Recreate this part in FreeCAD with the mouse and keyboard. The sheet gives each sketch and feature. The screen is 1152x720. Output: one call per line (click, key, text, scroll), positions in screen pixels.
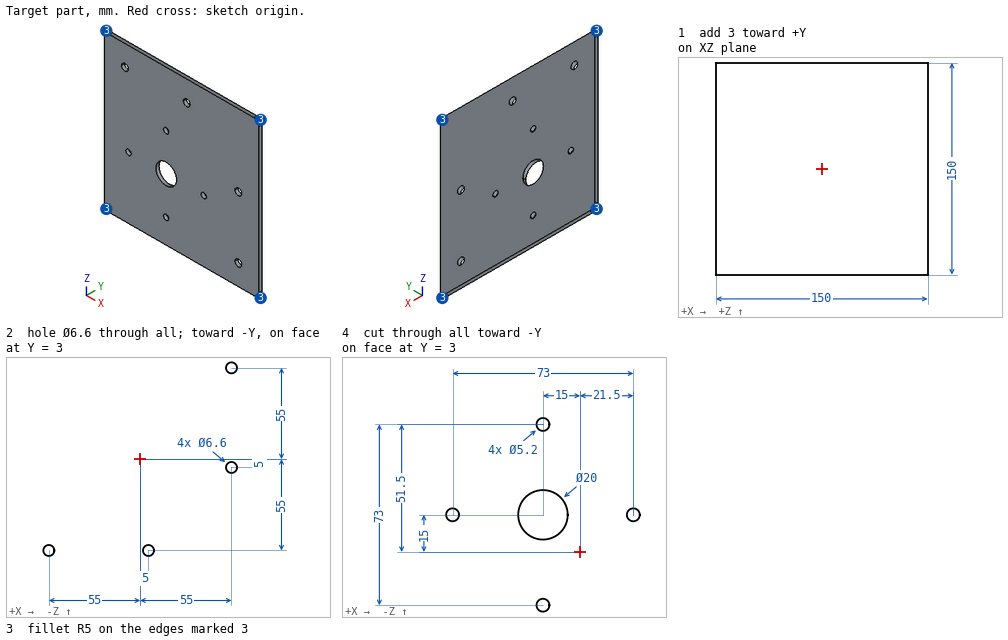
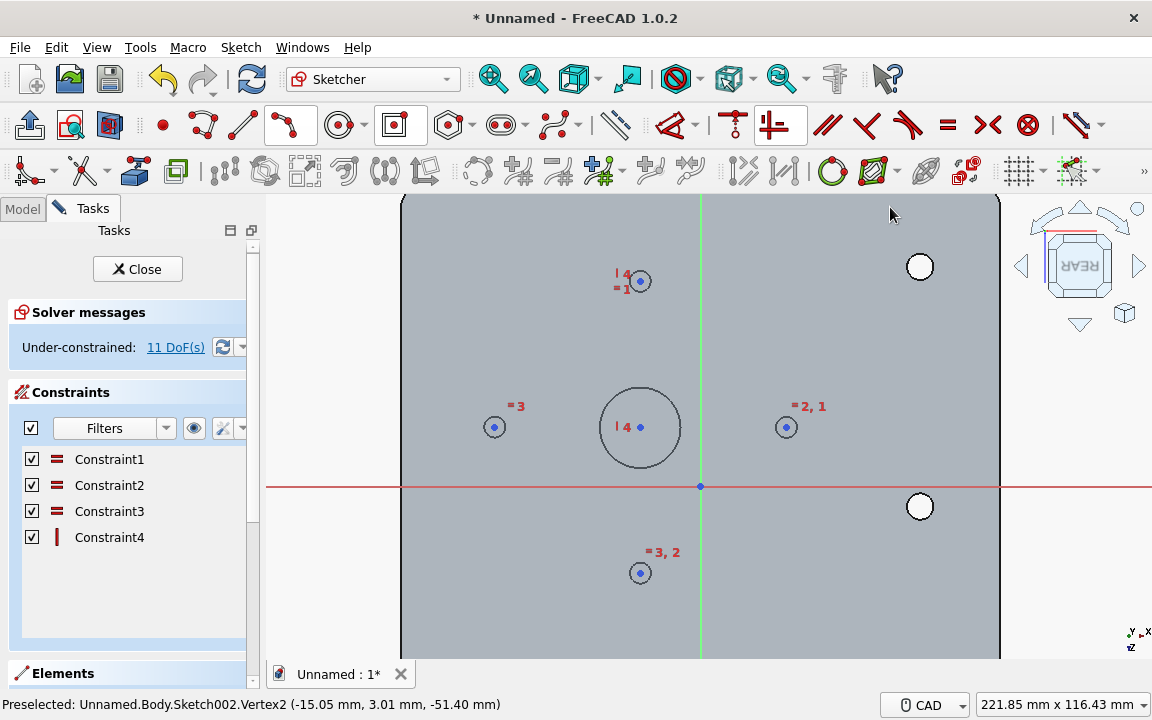
click(640, 428)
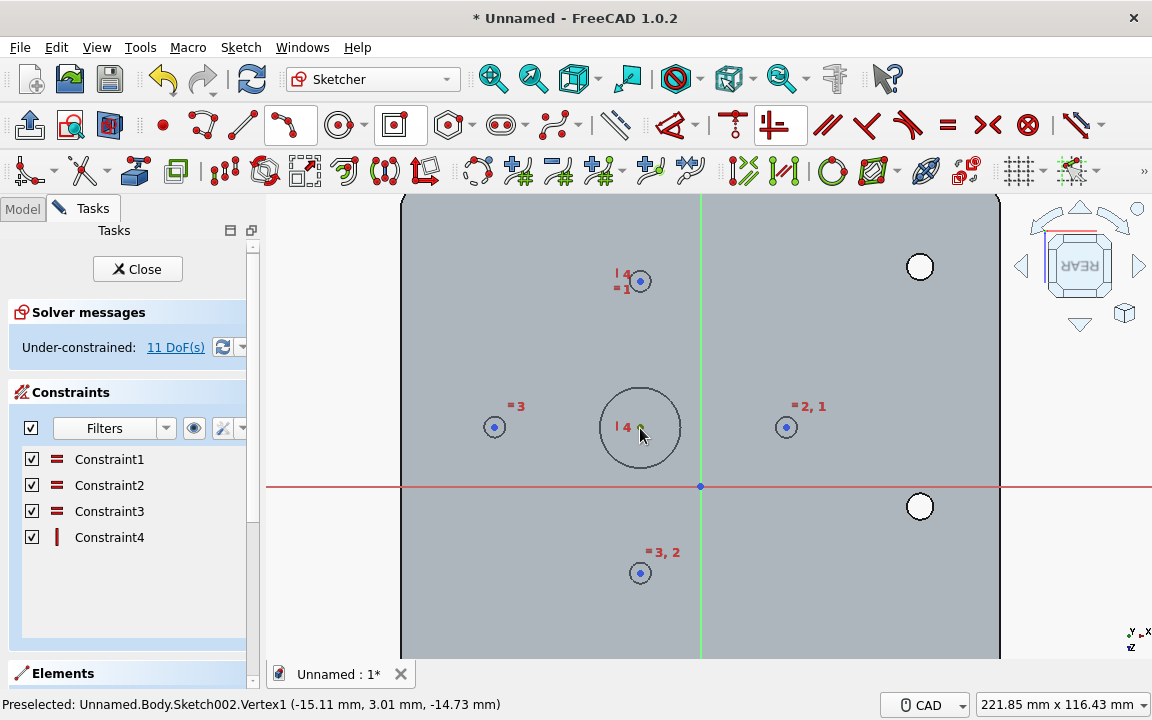
click(786, 427)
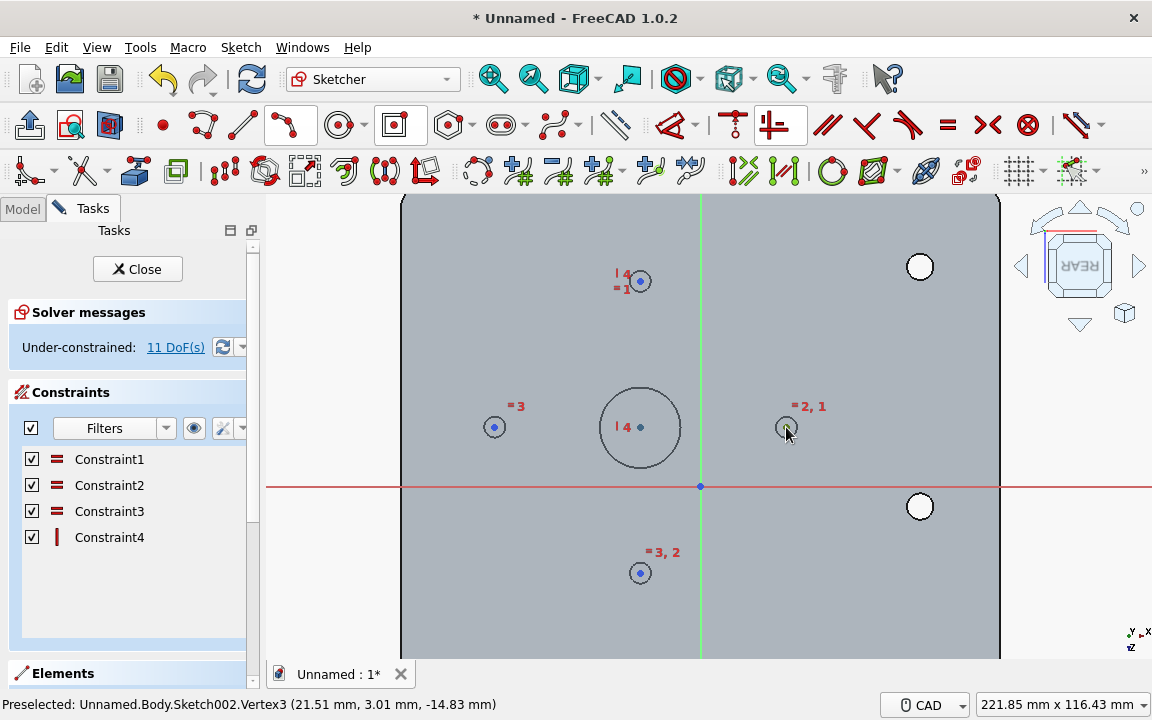
click(802, 126)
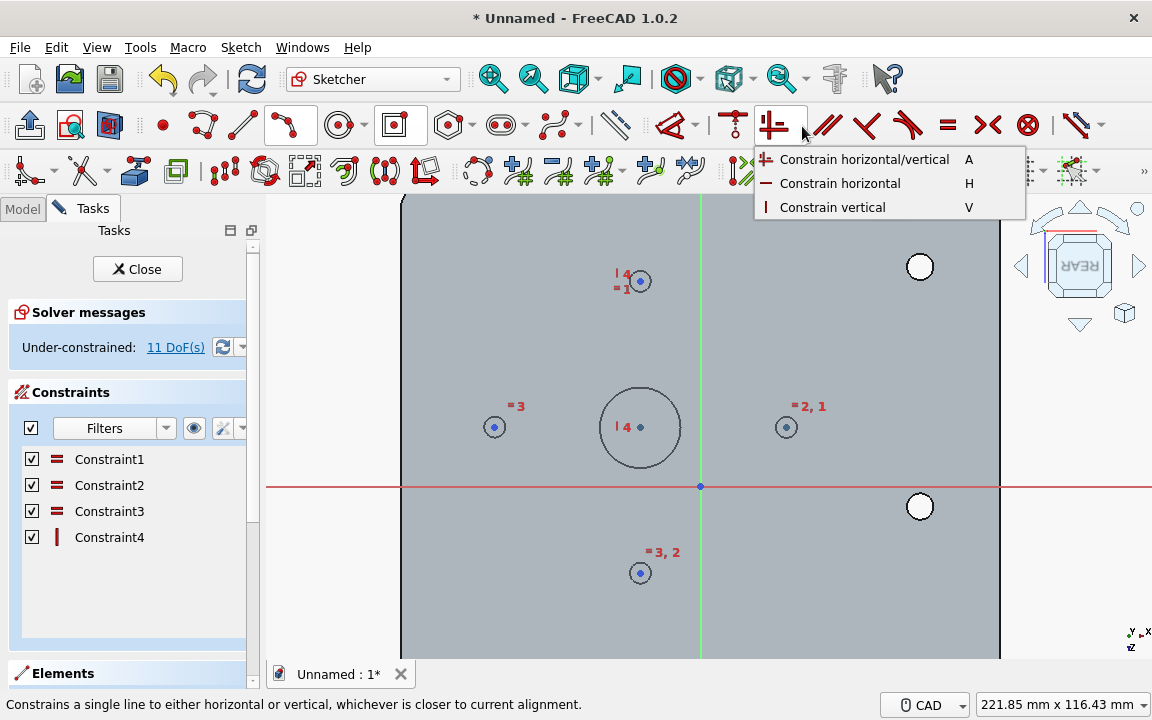
click(890, 183)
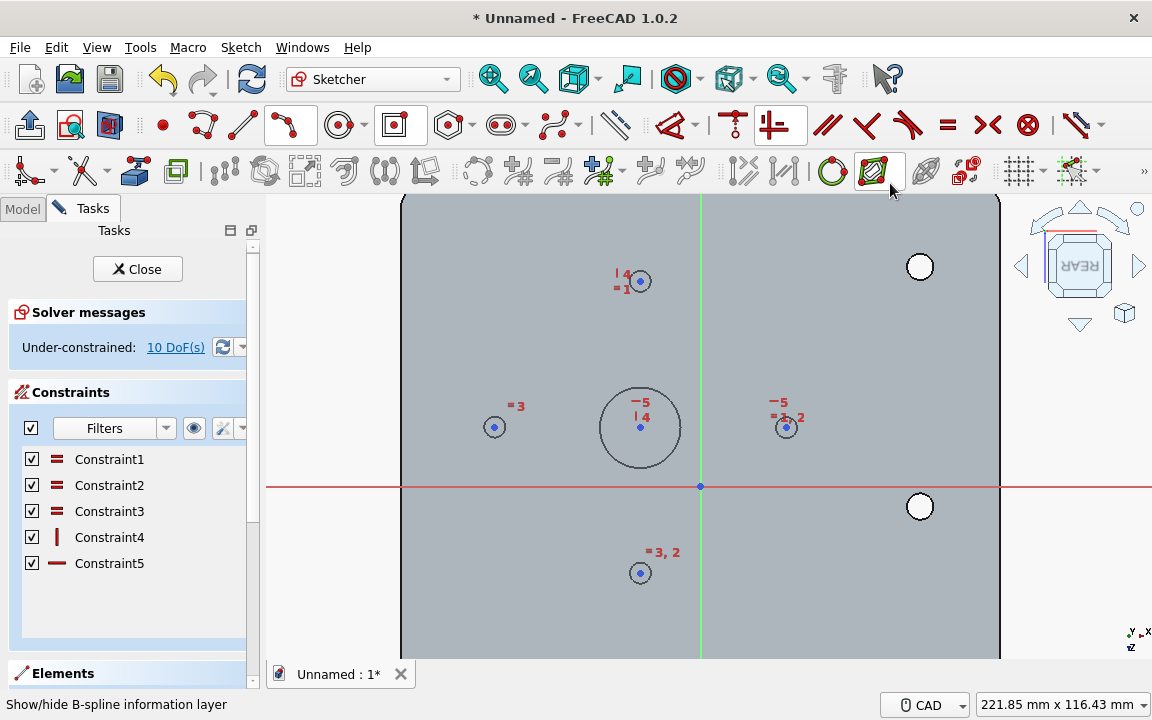
click(640, 428)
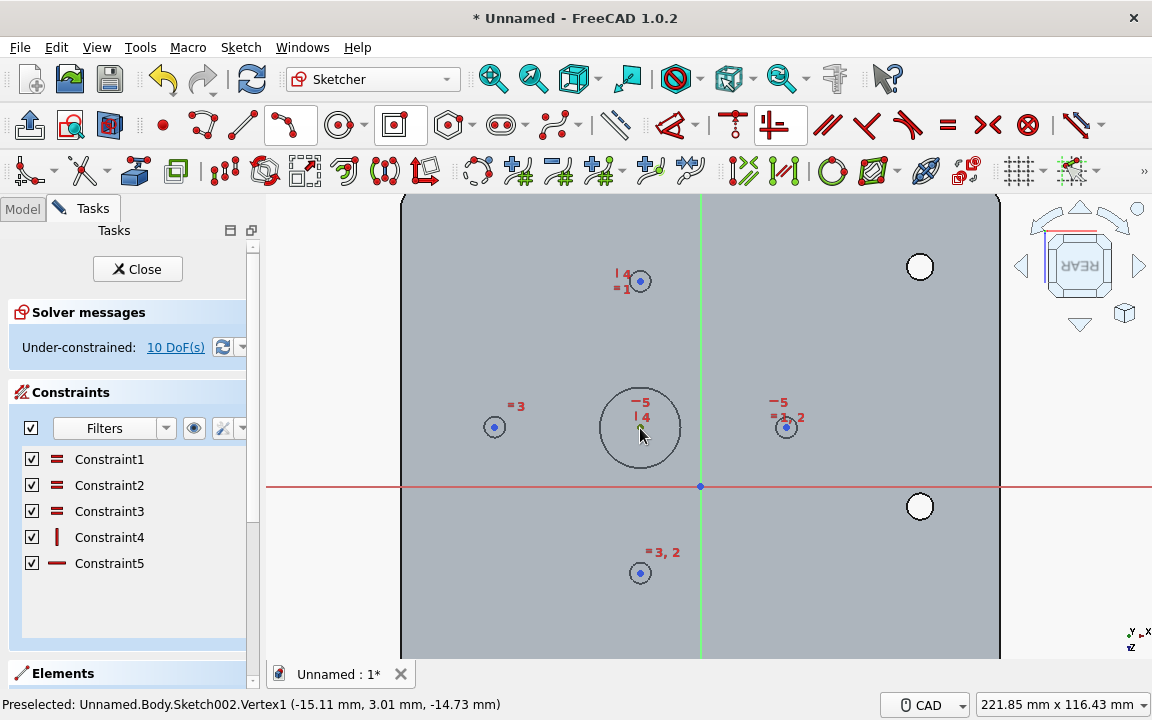
click(640, 573)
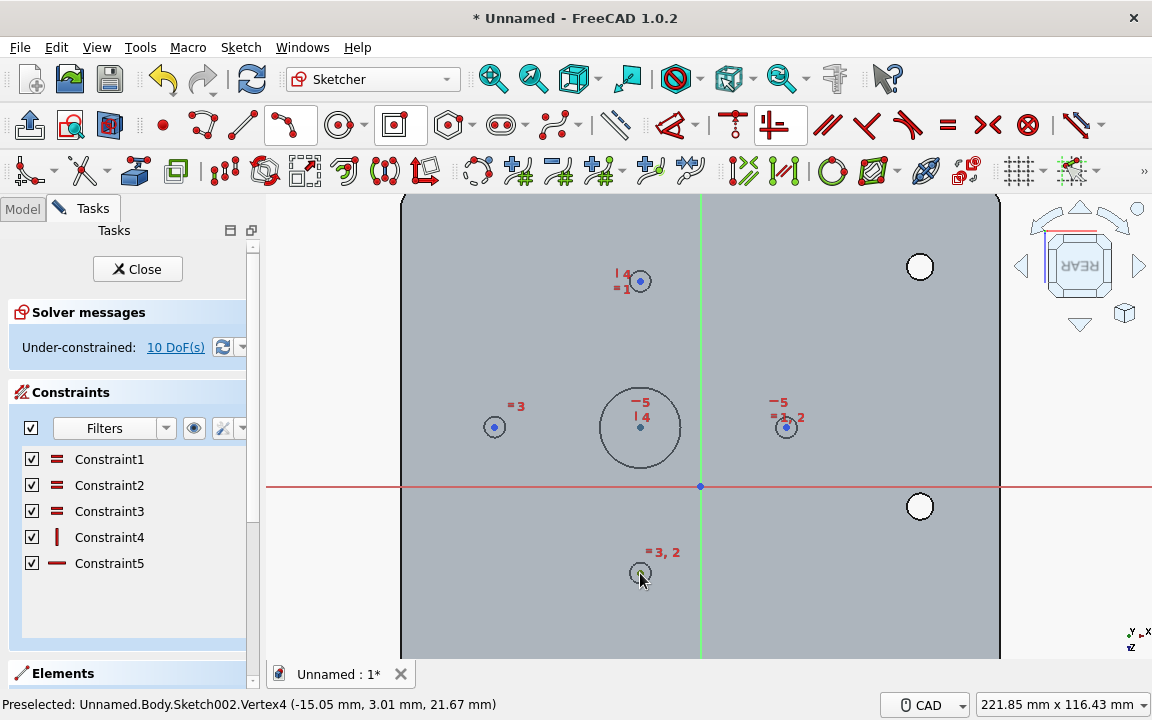
click(802, 126)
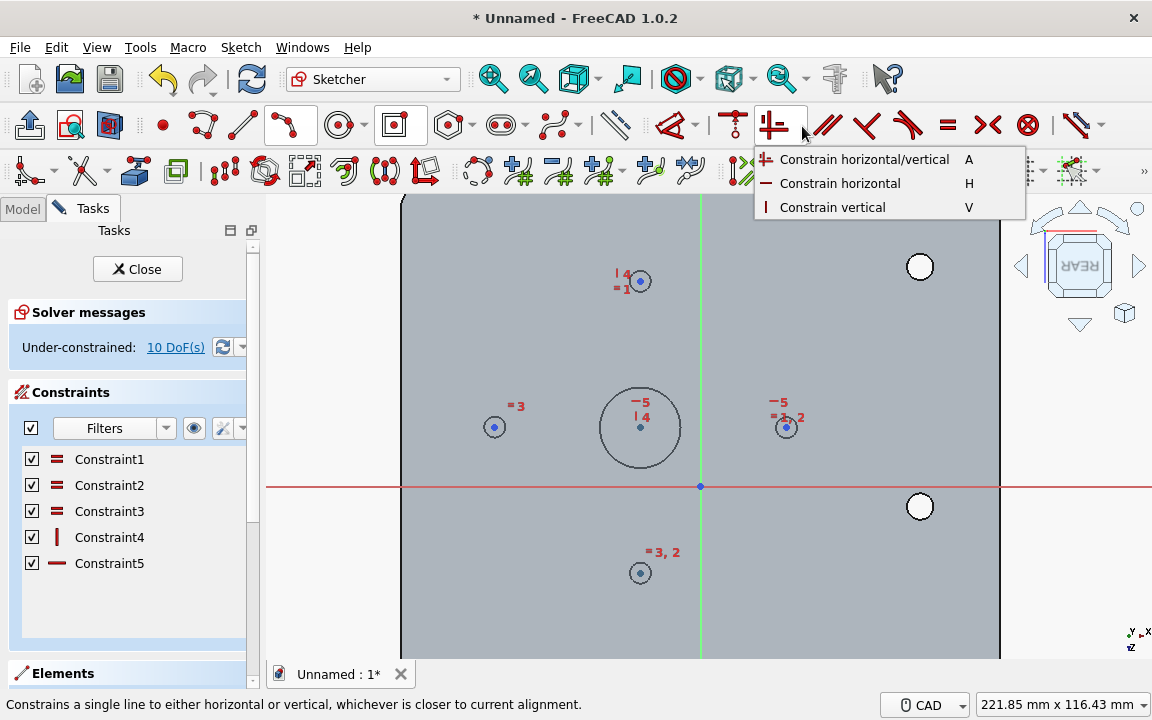
click(890, 207)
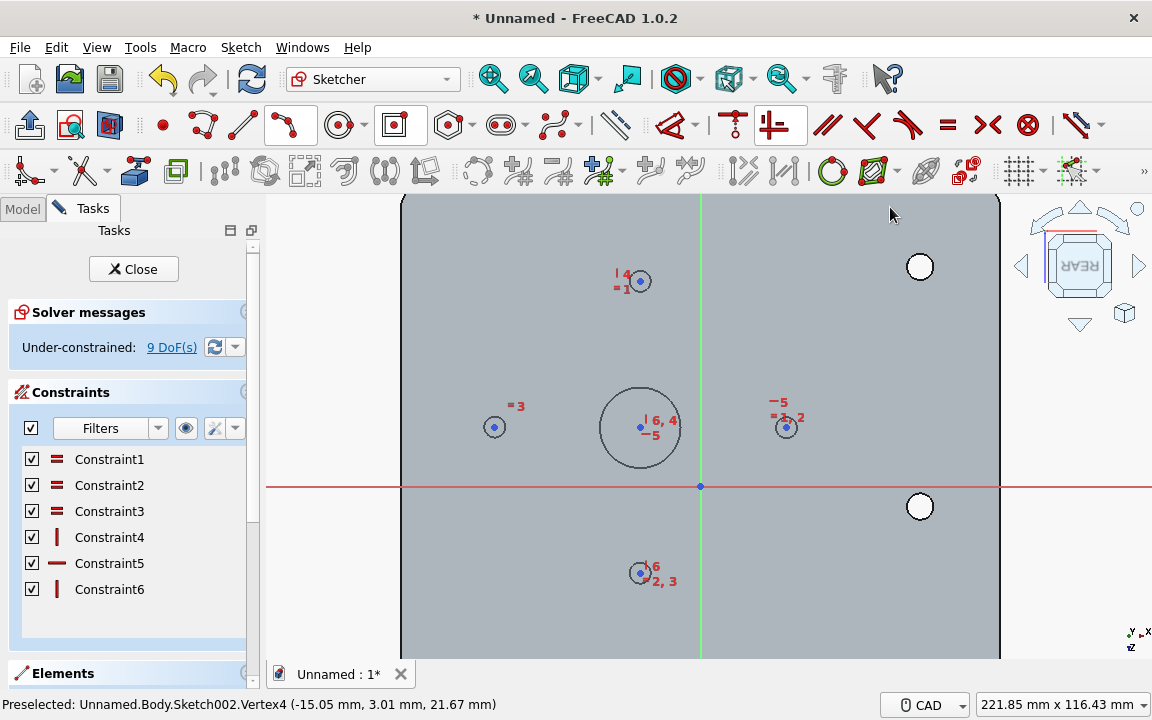
click(640, 428)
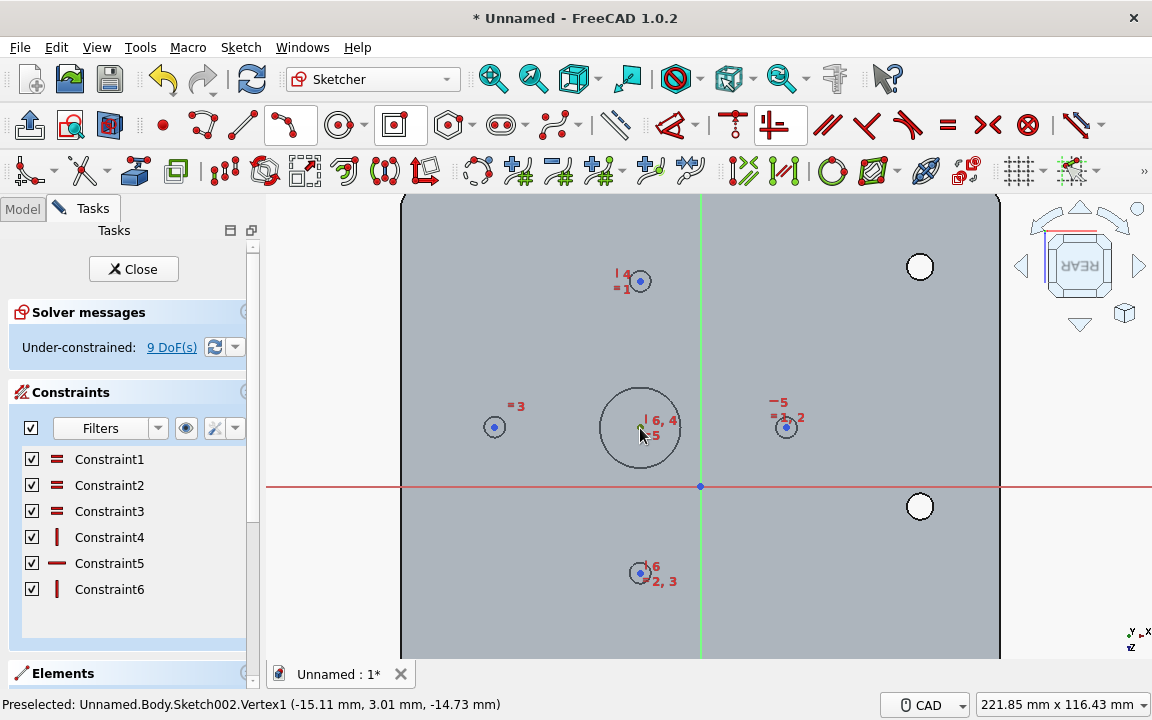
click(495, 427)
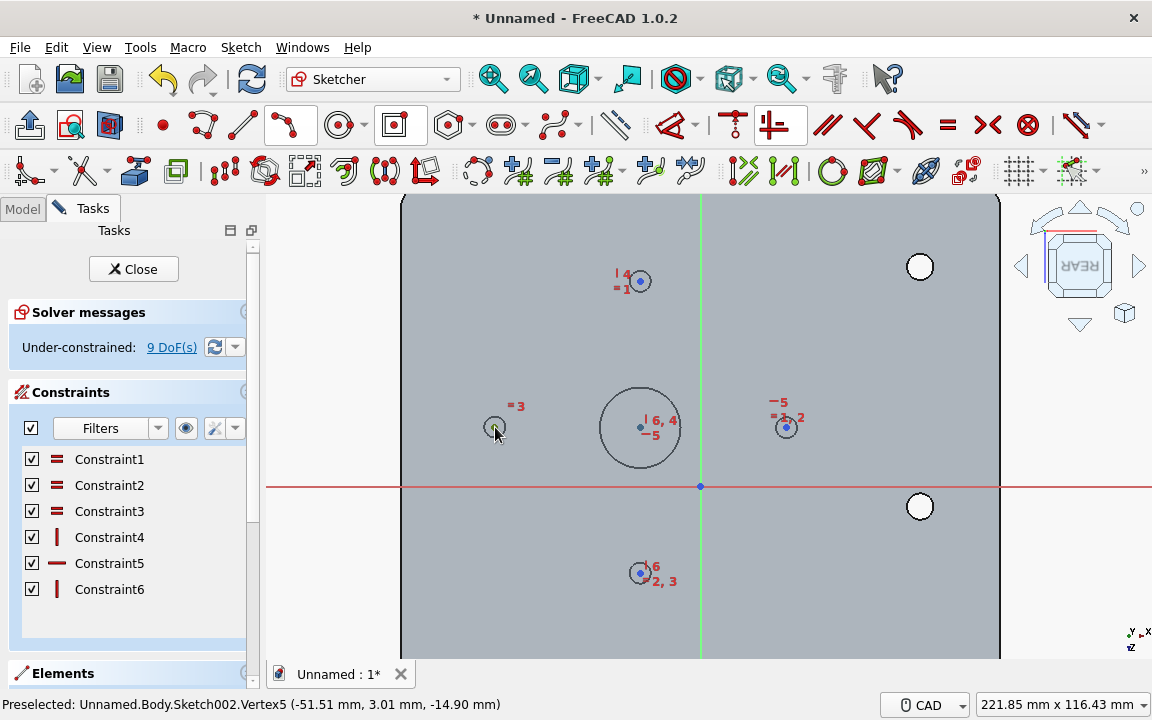
click(802, 126)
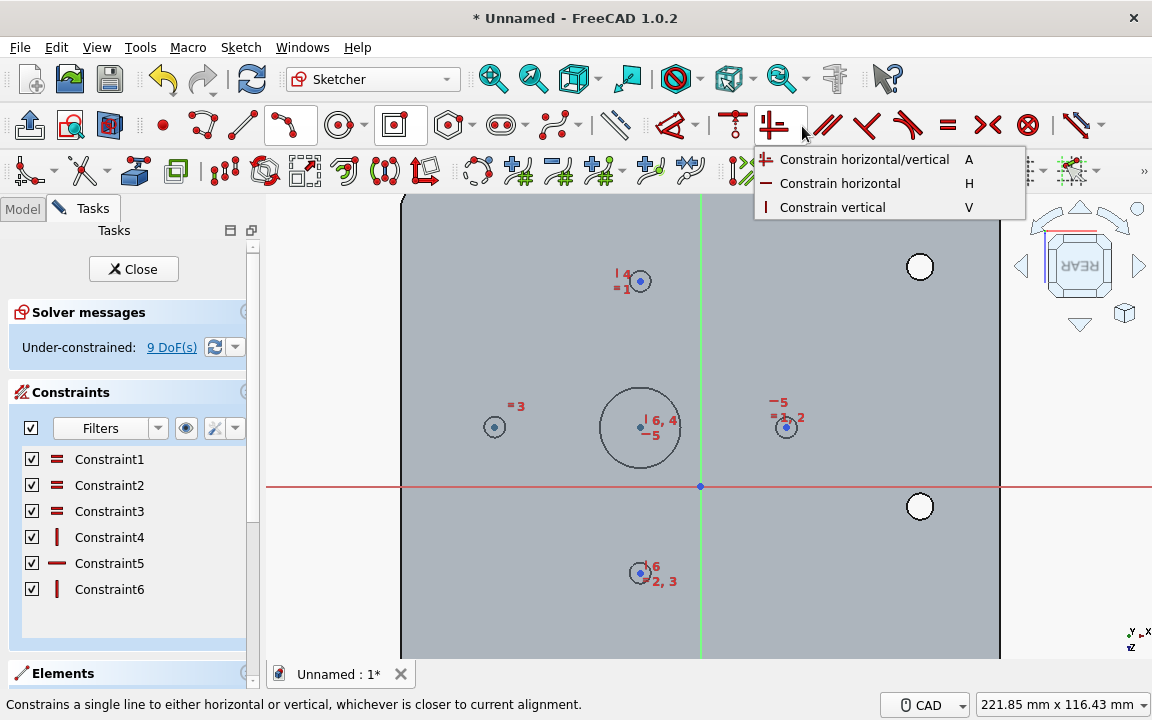
click(890, 183)